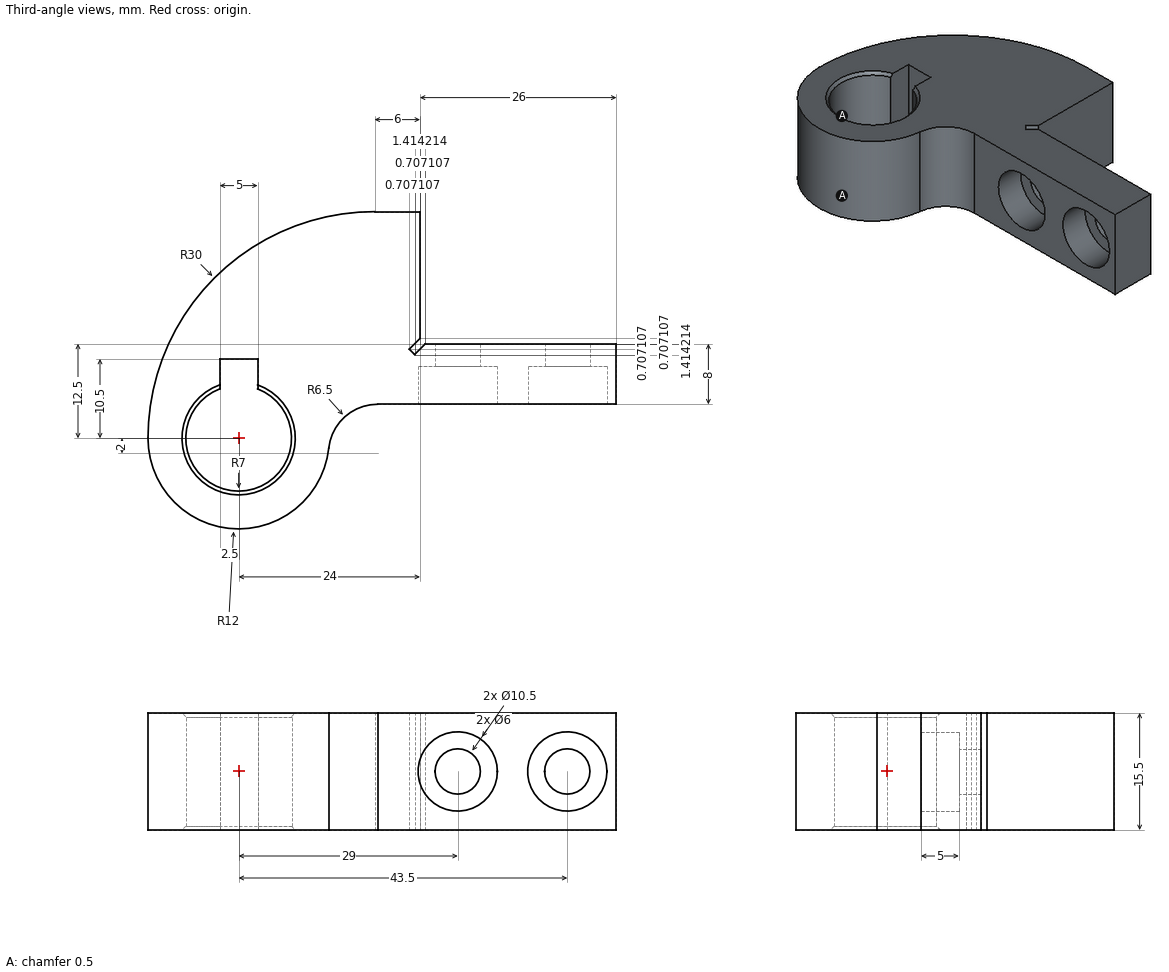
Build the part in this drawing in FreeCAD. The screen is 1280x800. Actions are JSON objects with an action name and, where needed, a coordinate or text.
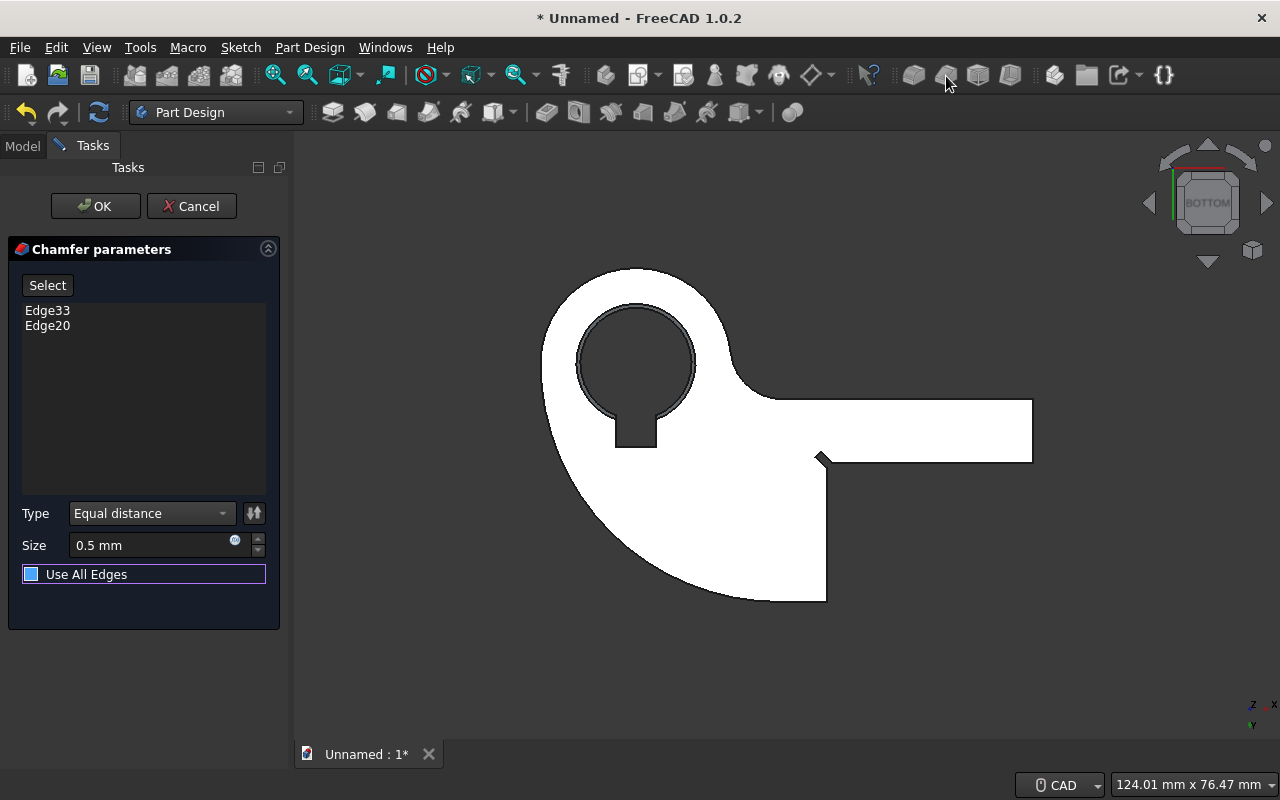
{"action": "left_click", "coordinate": [96, 206]}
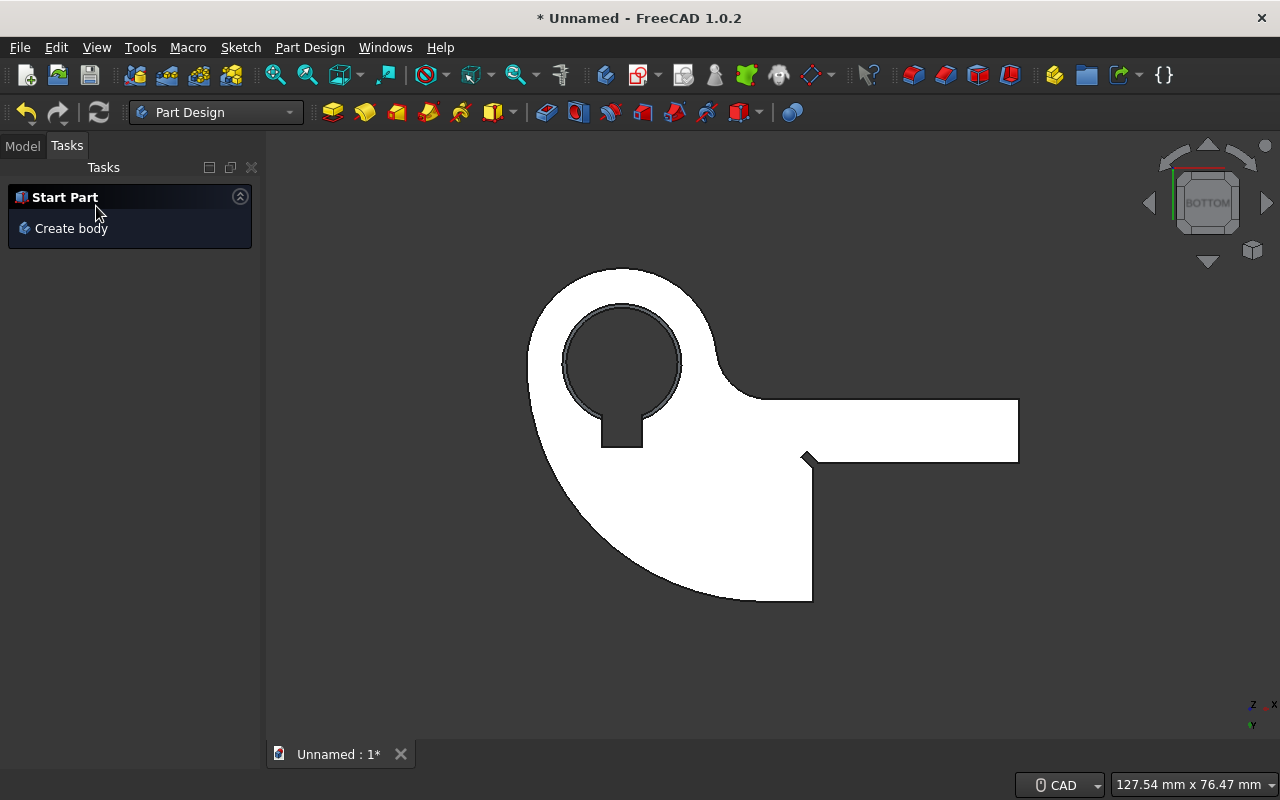
{"action": "key", "text": "0"}